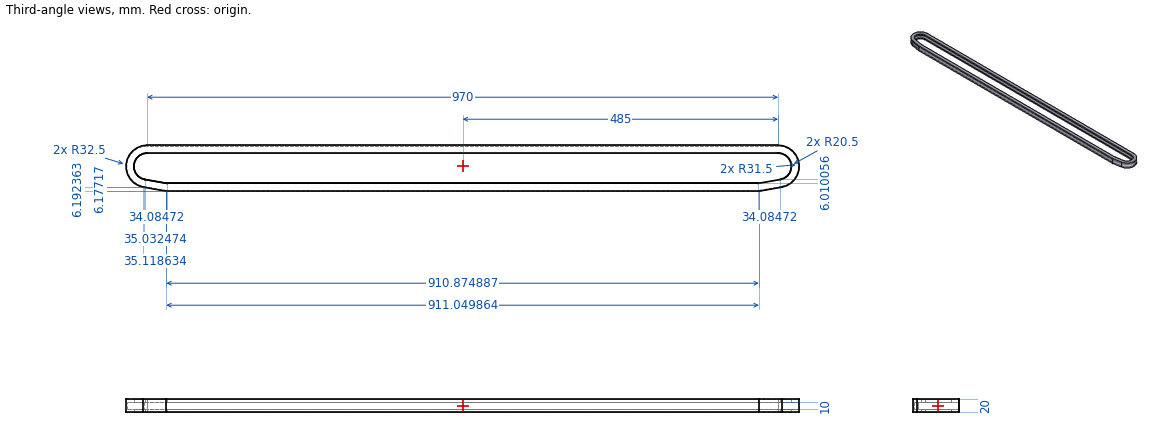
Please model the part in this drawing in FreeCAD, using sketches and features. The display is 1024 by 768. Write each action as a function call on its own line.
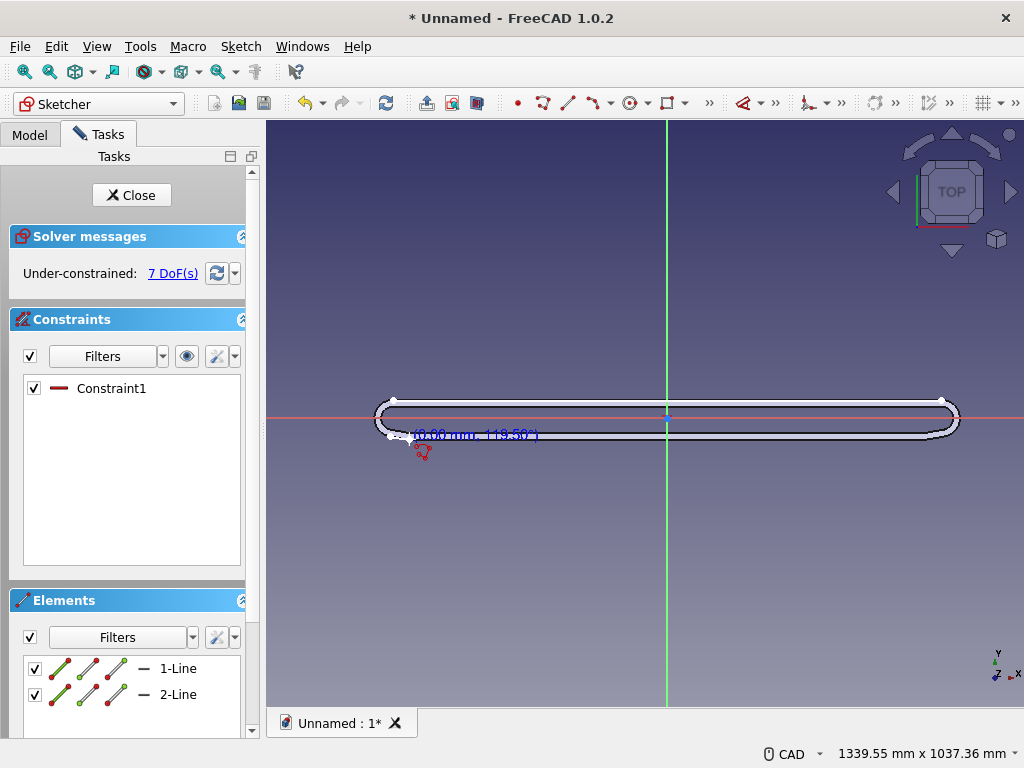
scroll(392, 400, down, 2)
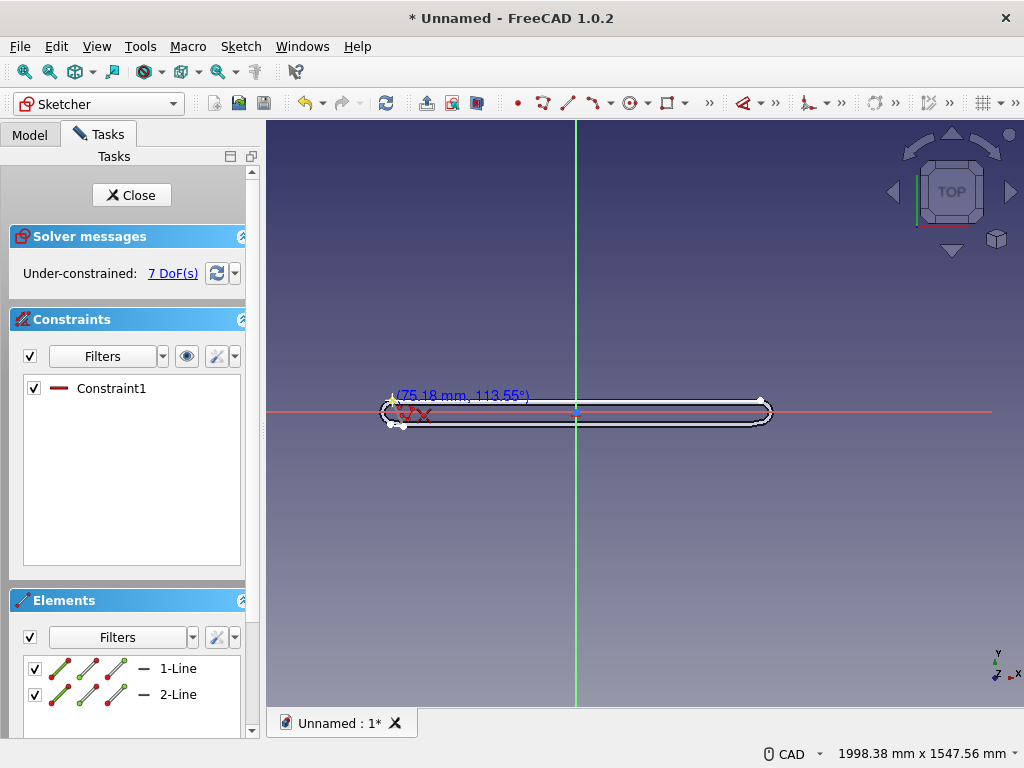
click(749, 426)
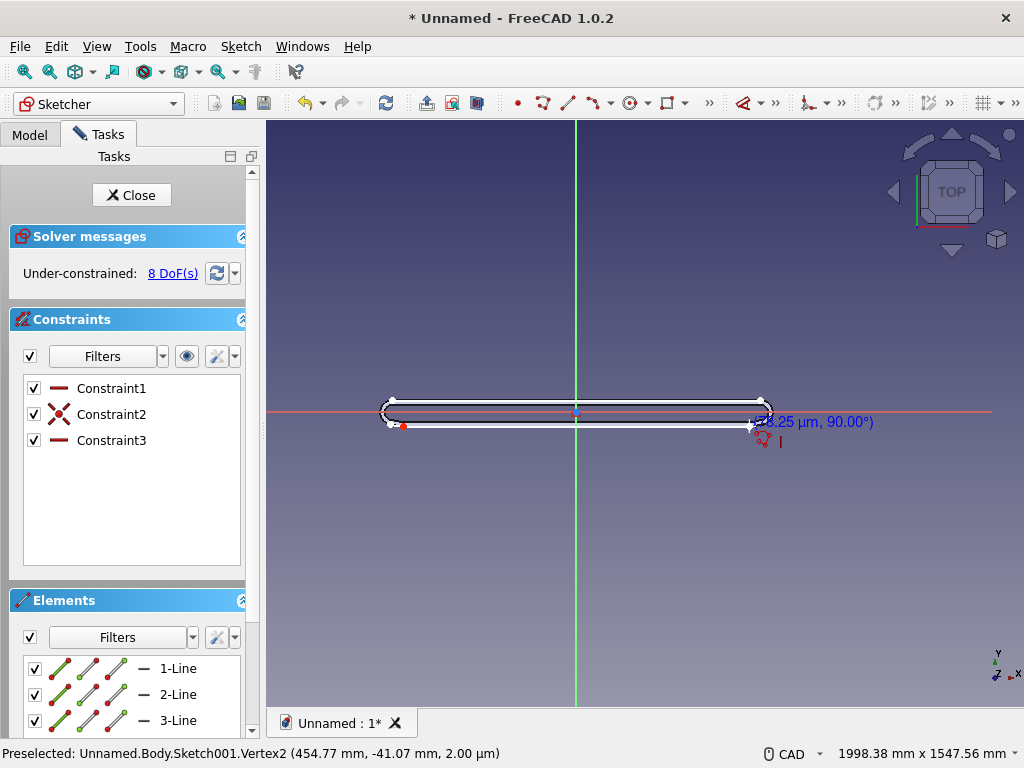
scroll(763, 424, up, 2)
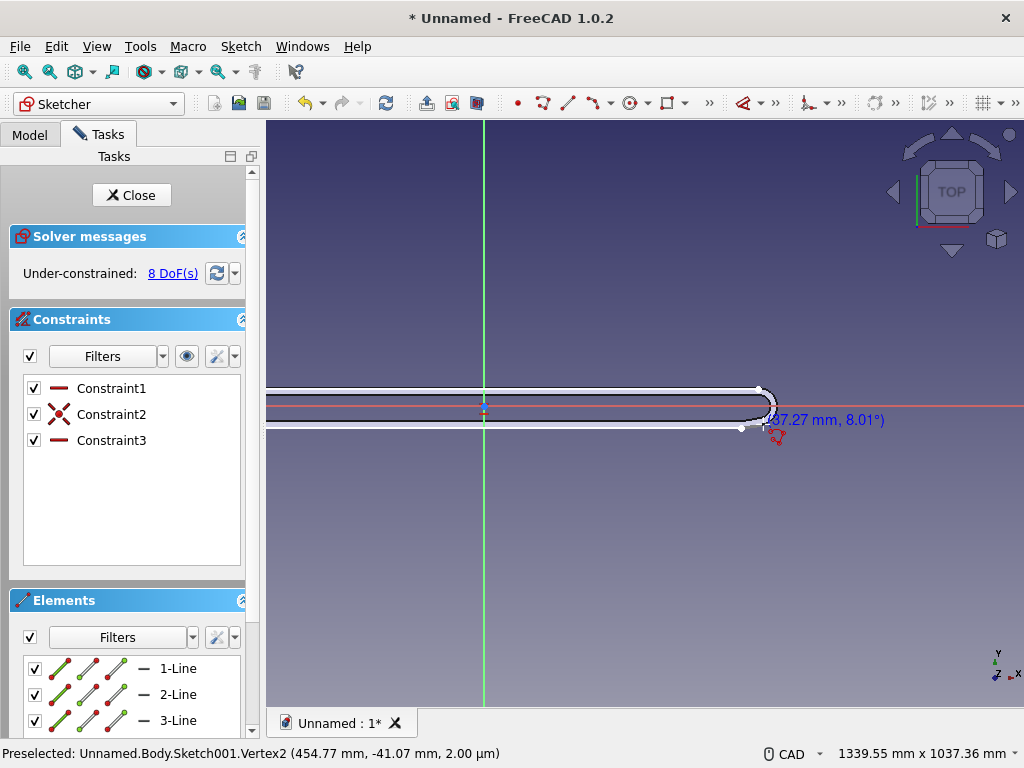
click(762, 424)
right_click(762, 424)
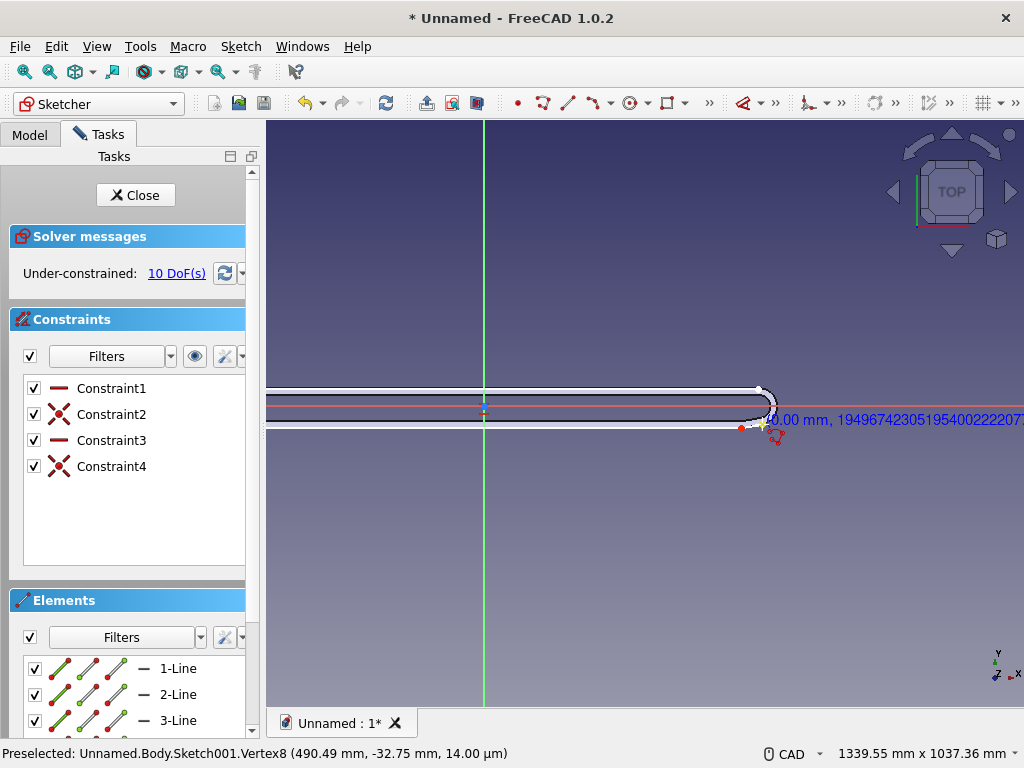
key(g)
key(3)
key(a)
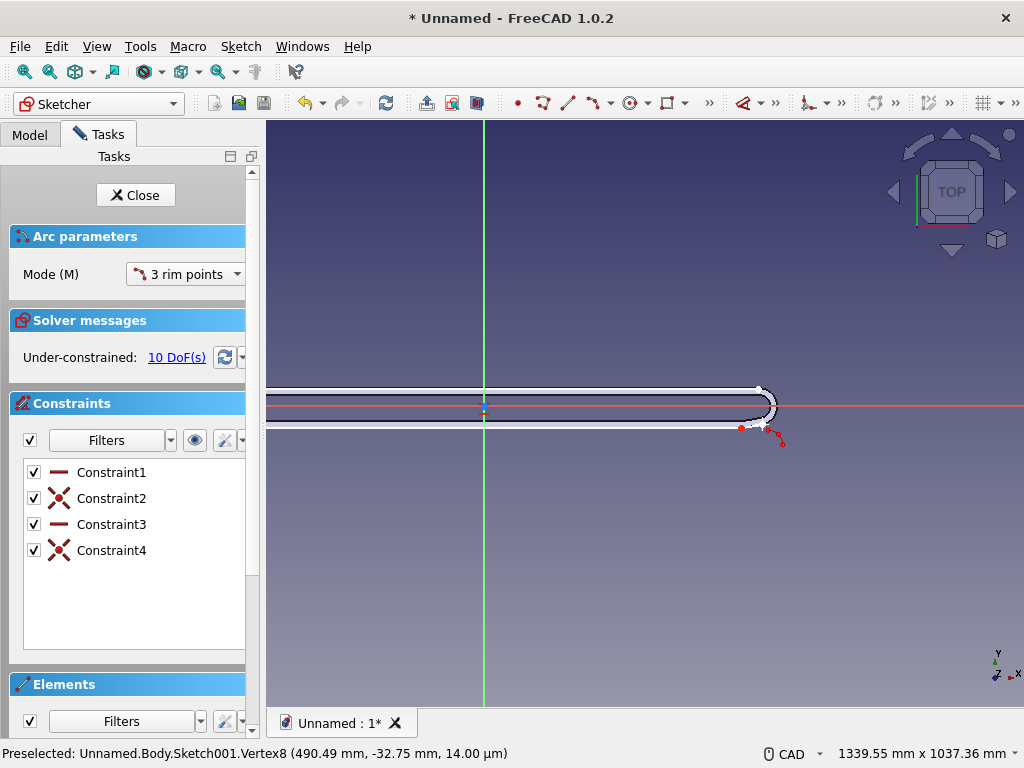
scroll(764, 425, down, 2)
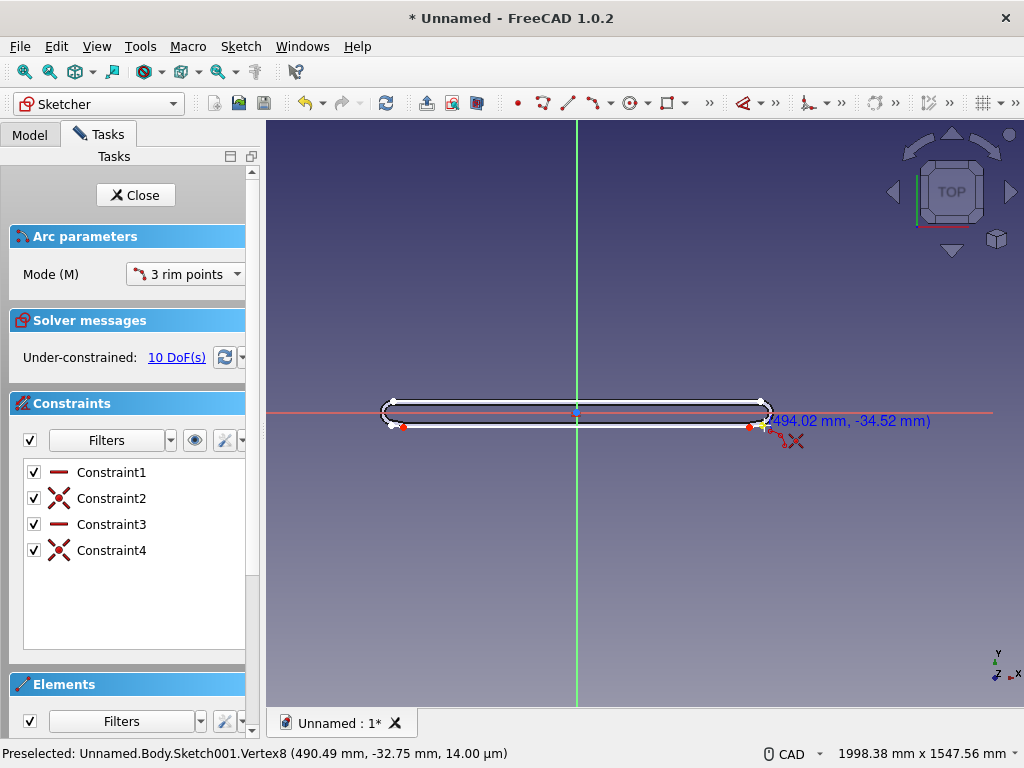
scroll(393, 401, up, 2)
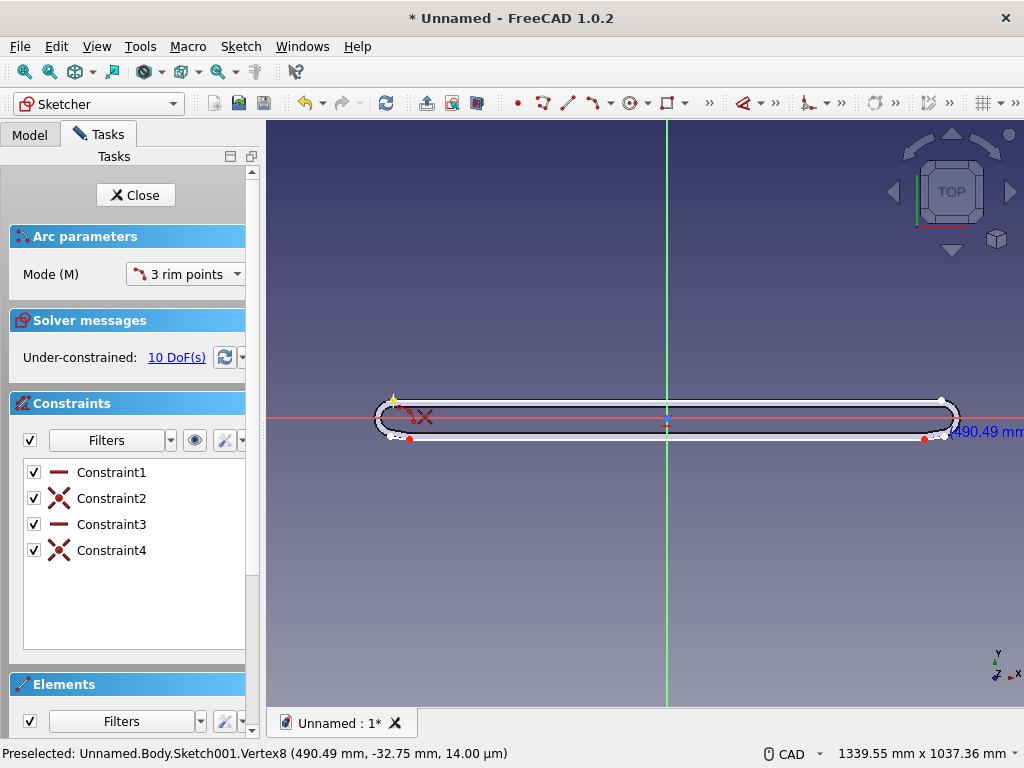
click(393, 401)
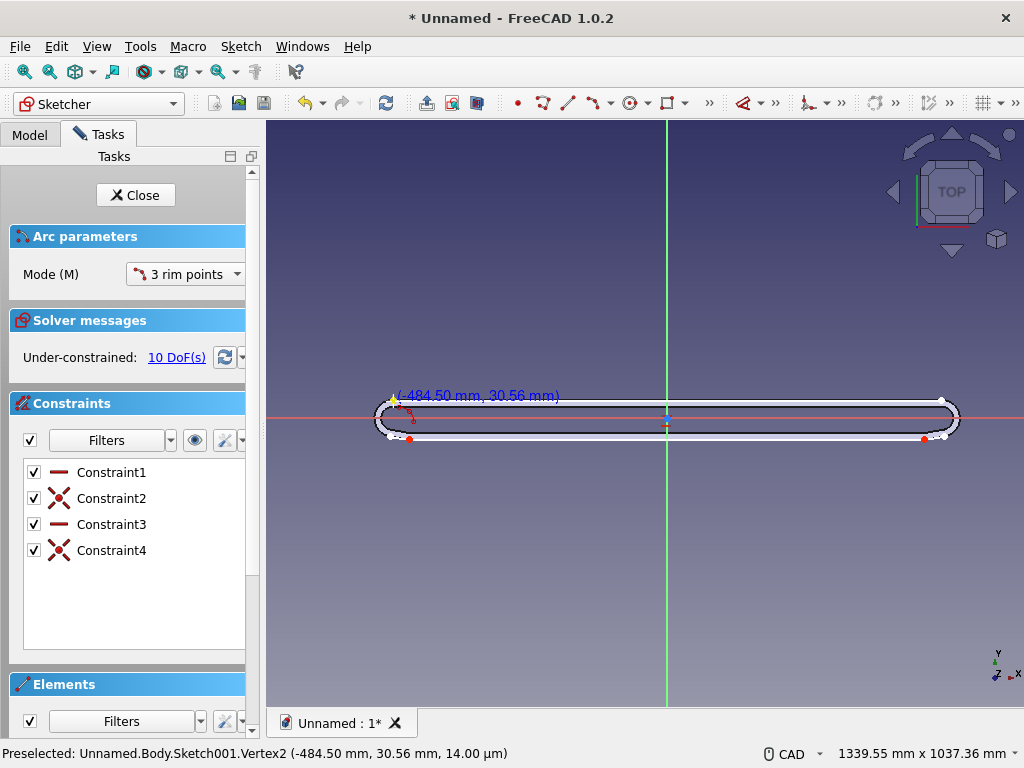
scroll(390, 436, up, 3)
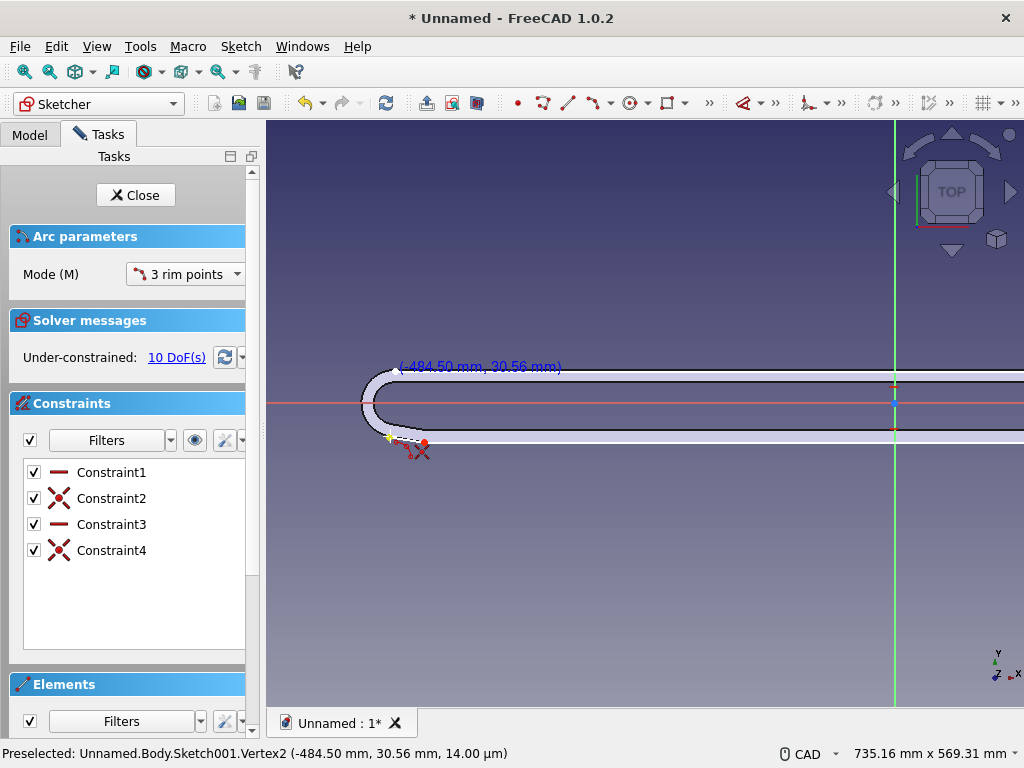
click(390, 437)
click(370, 383)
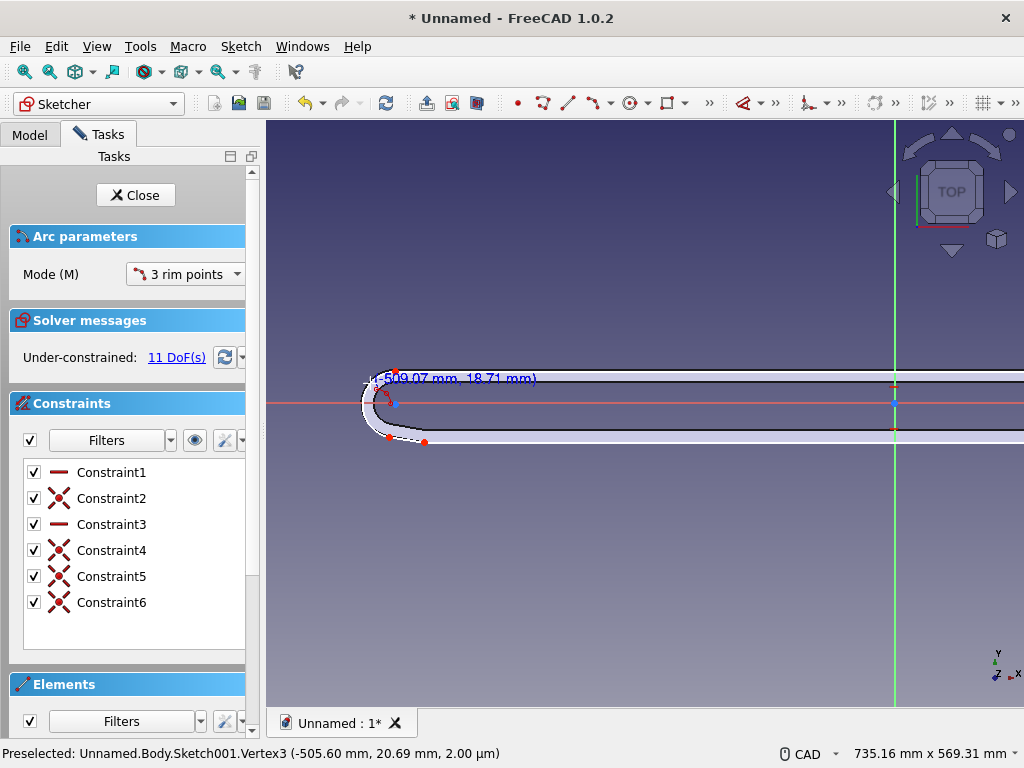
scroll(391, 418, down, 5)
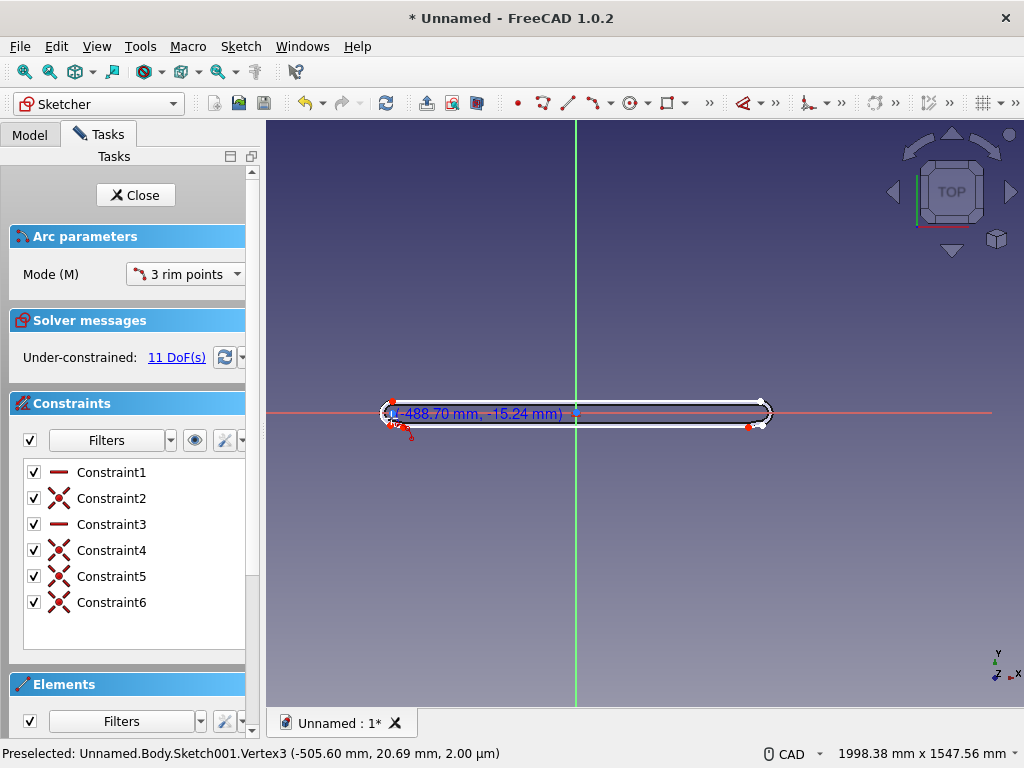
scroll(763, 425, up, 5)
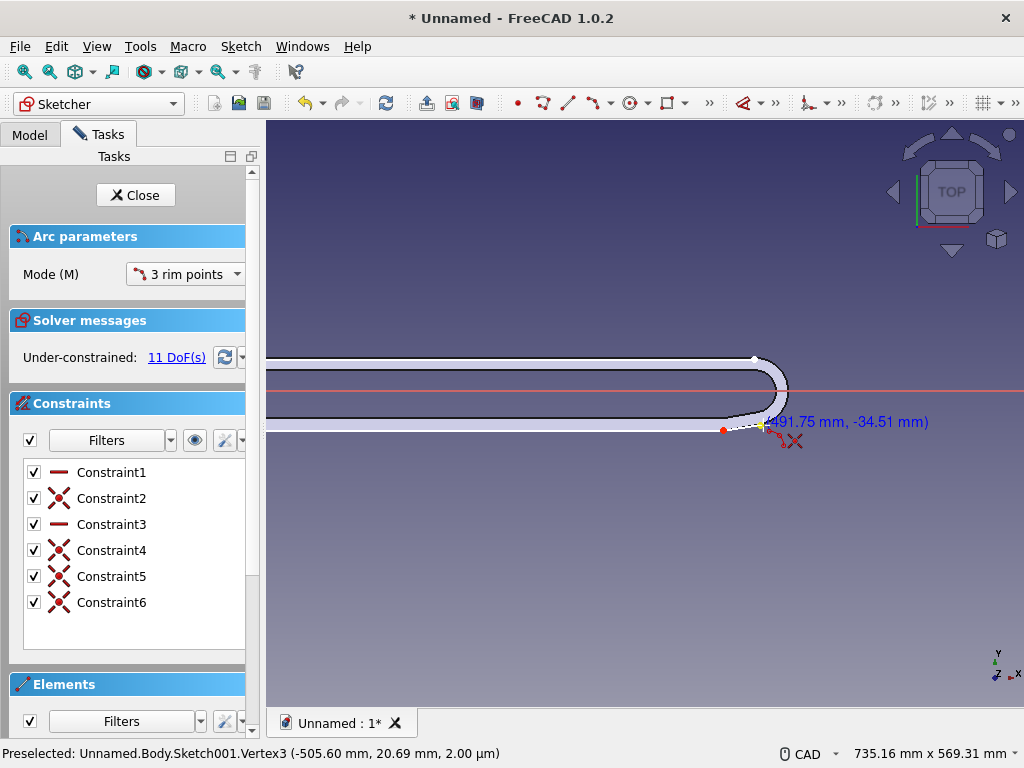
click(761, 425)
click(754, 360)
click(780, 371)
key(Escape)